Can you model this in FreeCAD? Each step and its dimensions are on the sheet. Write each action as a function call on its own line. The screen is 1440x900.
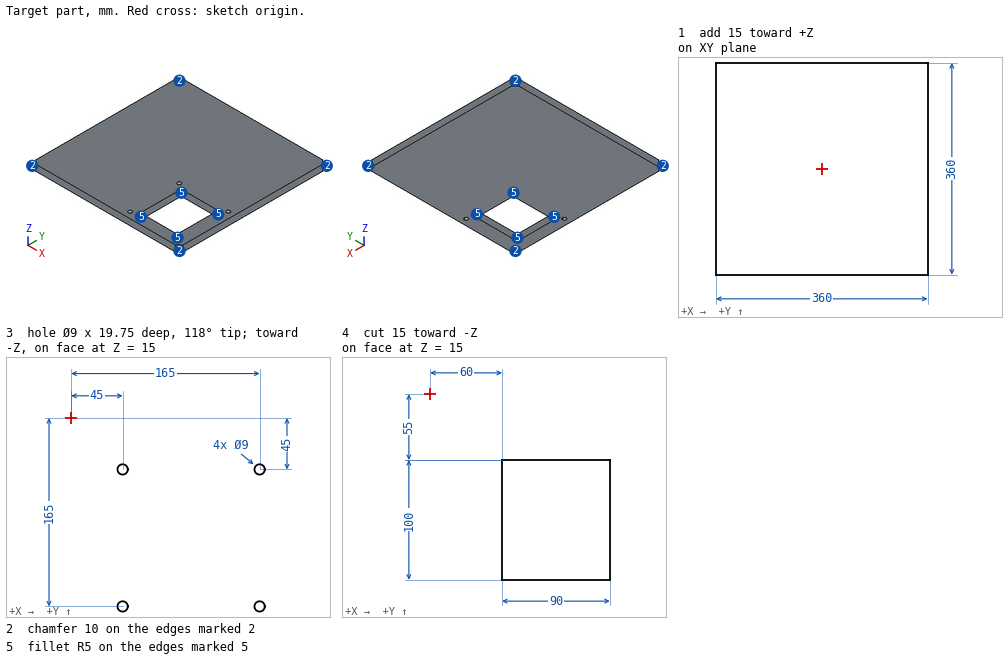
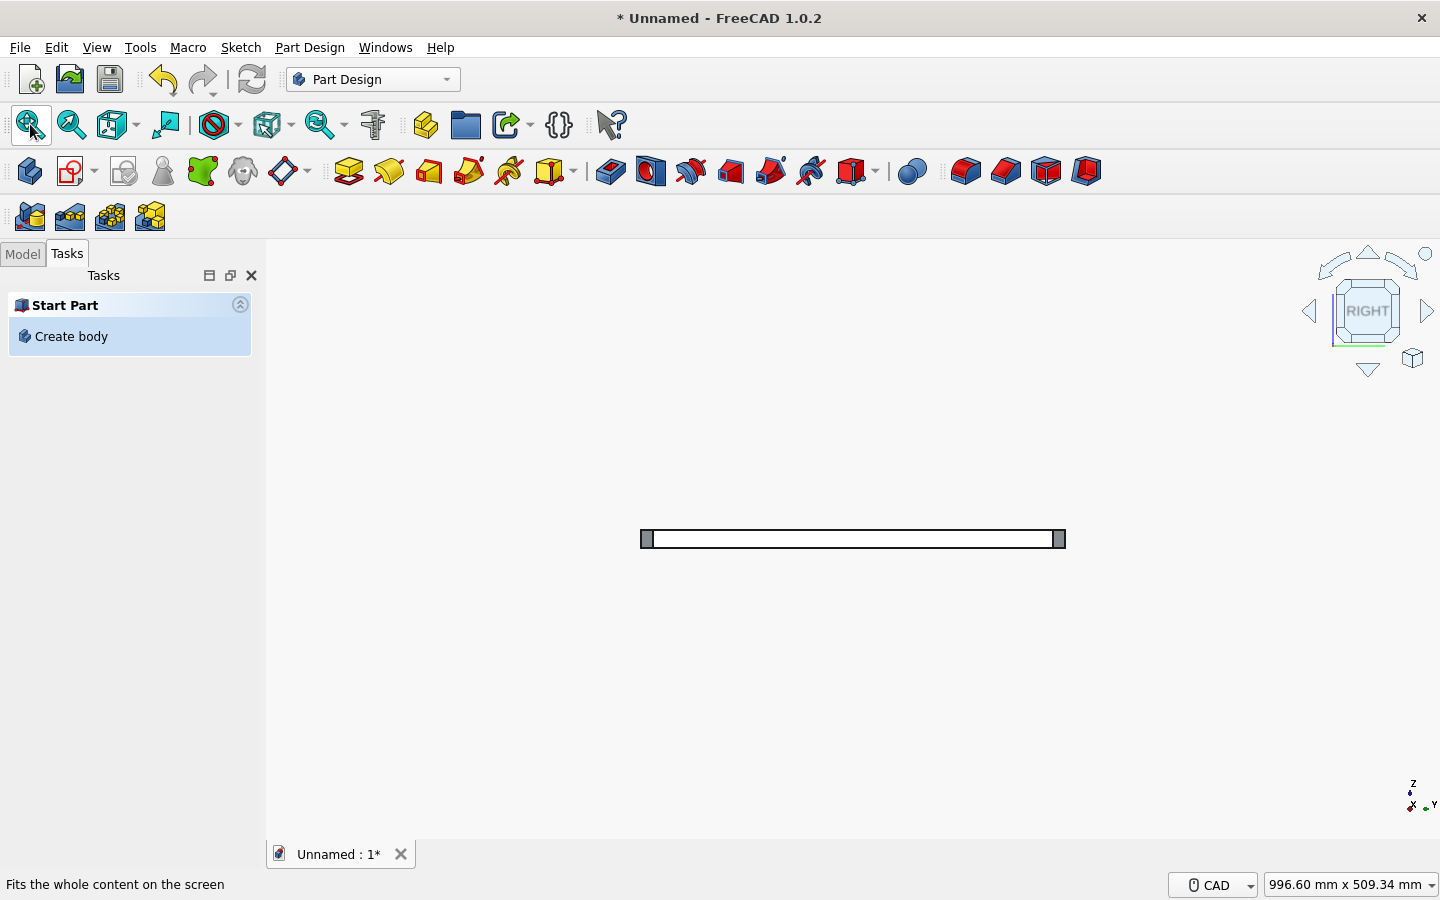
scroll(788, 538, up, 5)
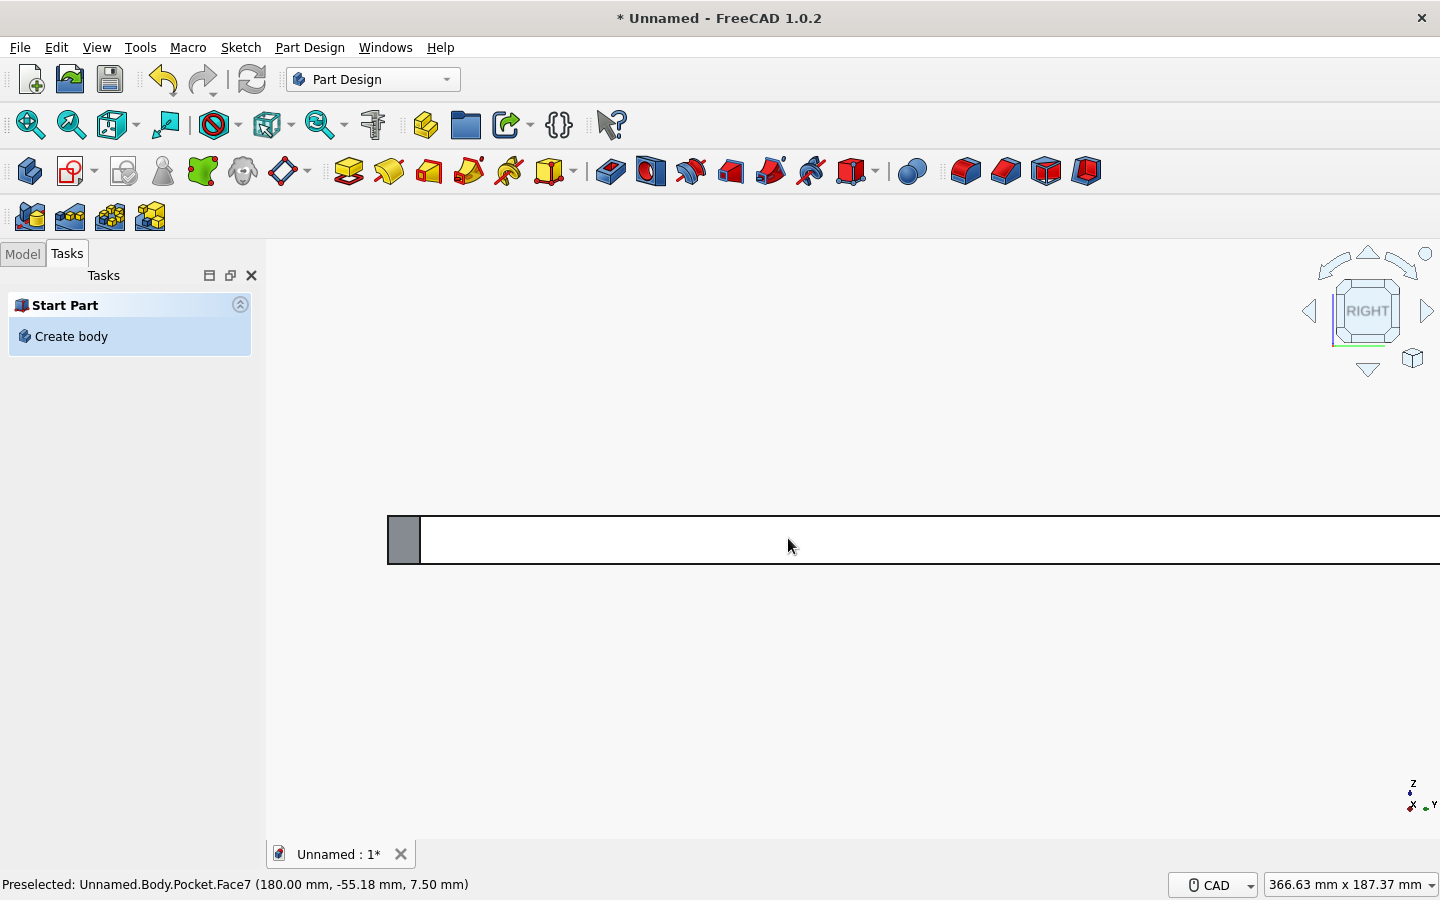
key(v)
key(f)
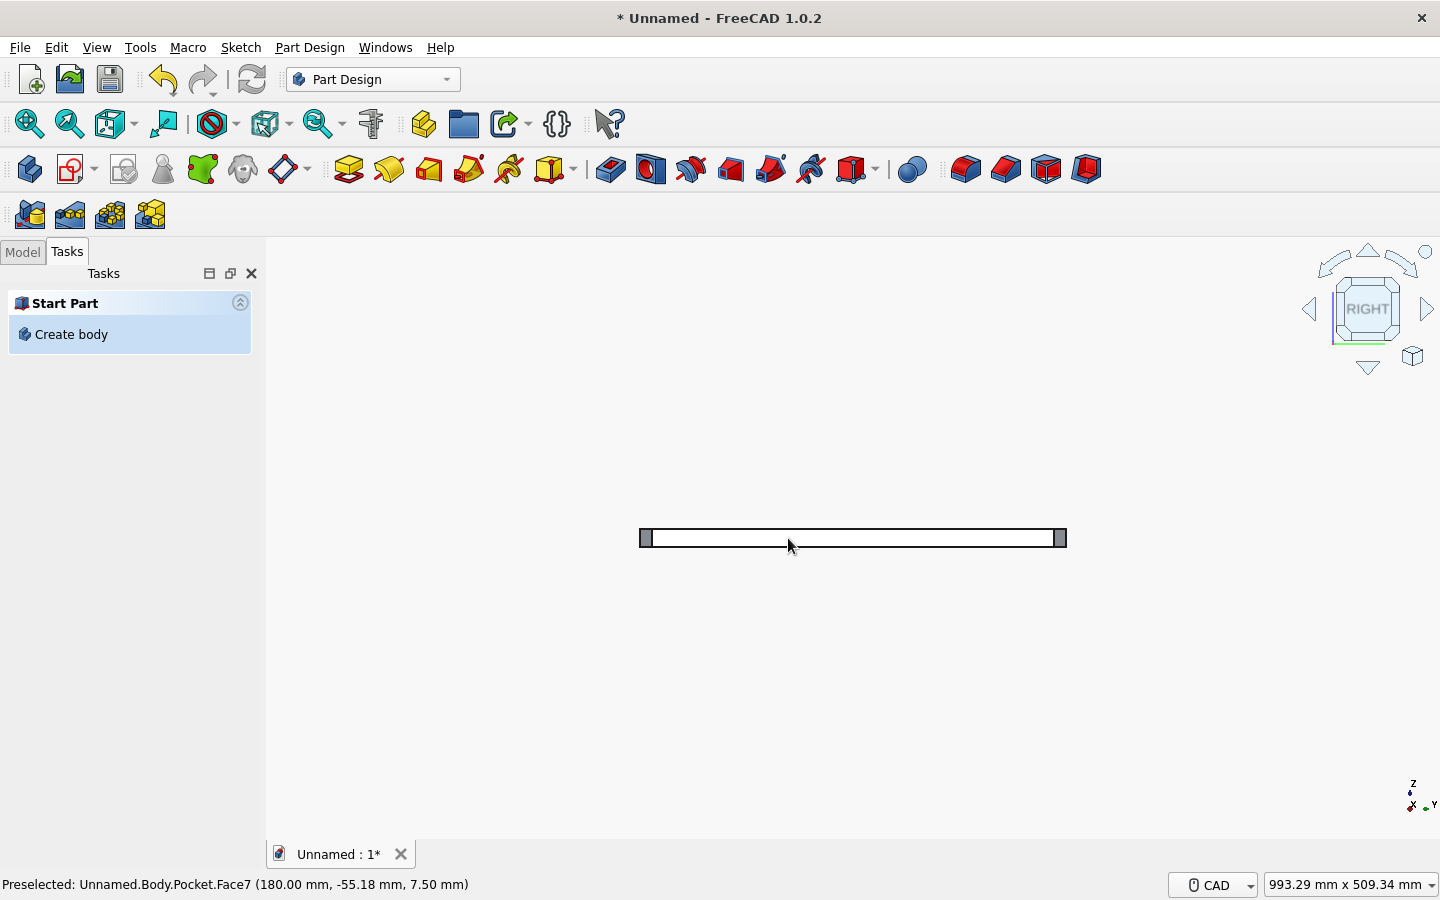
key(5)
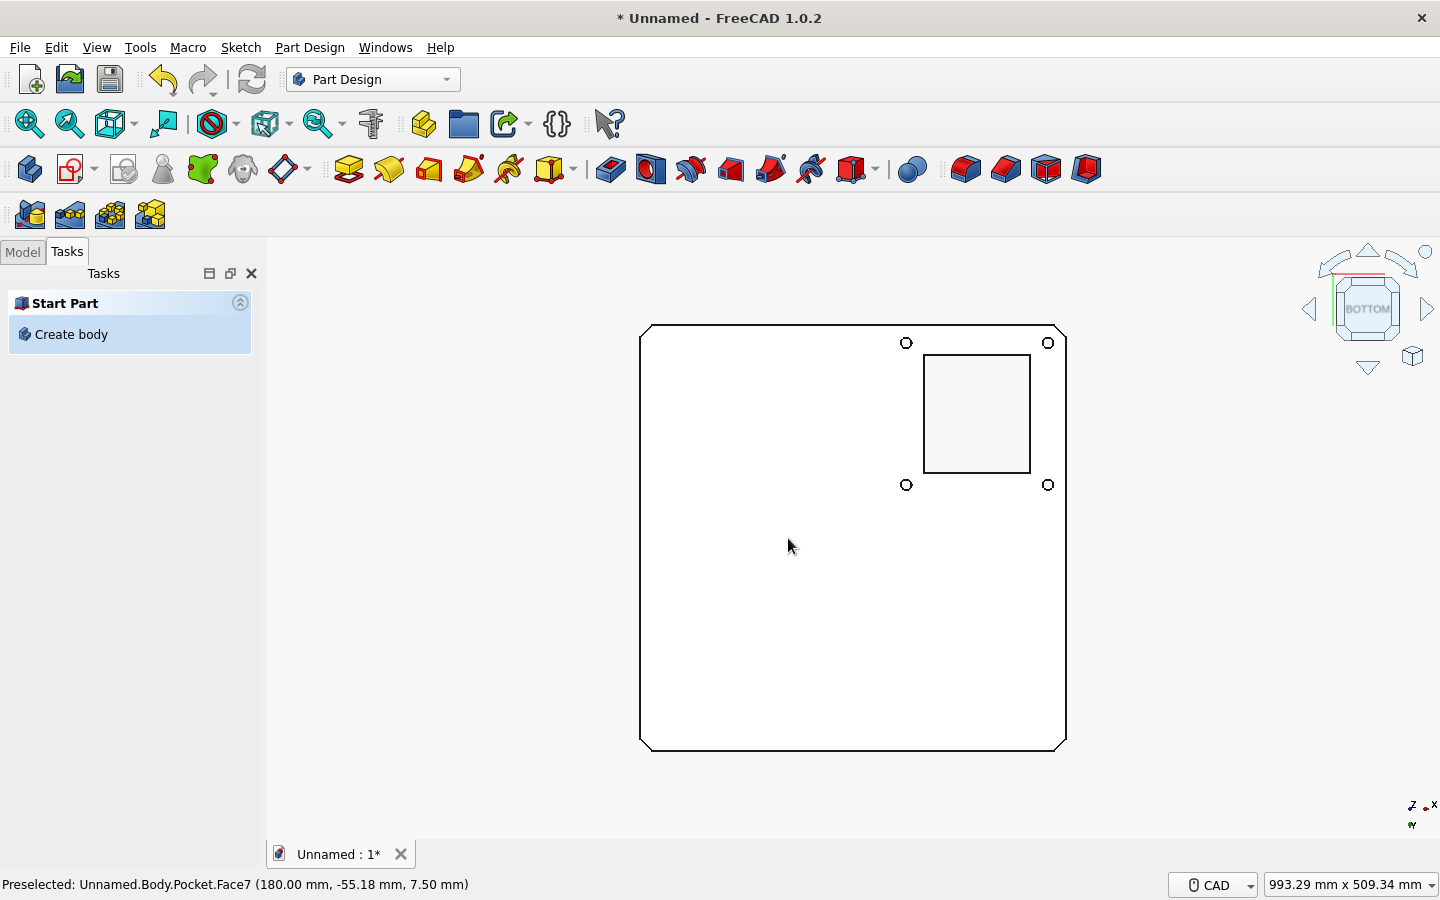
scroll(1030, 472, up, 5)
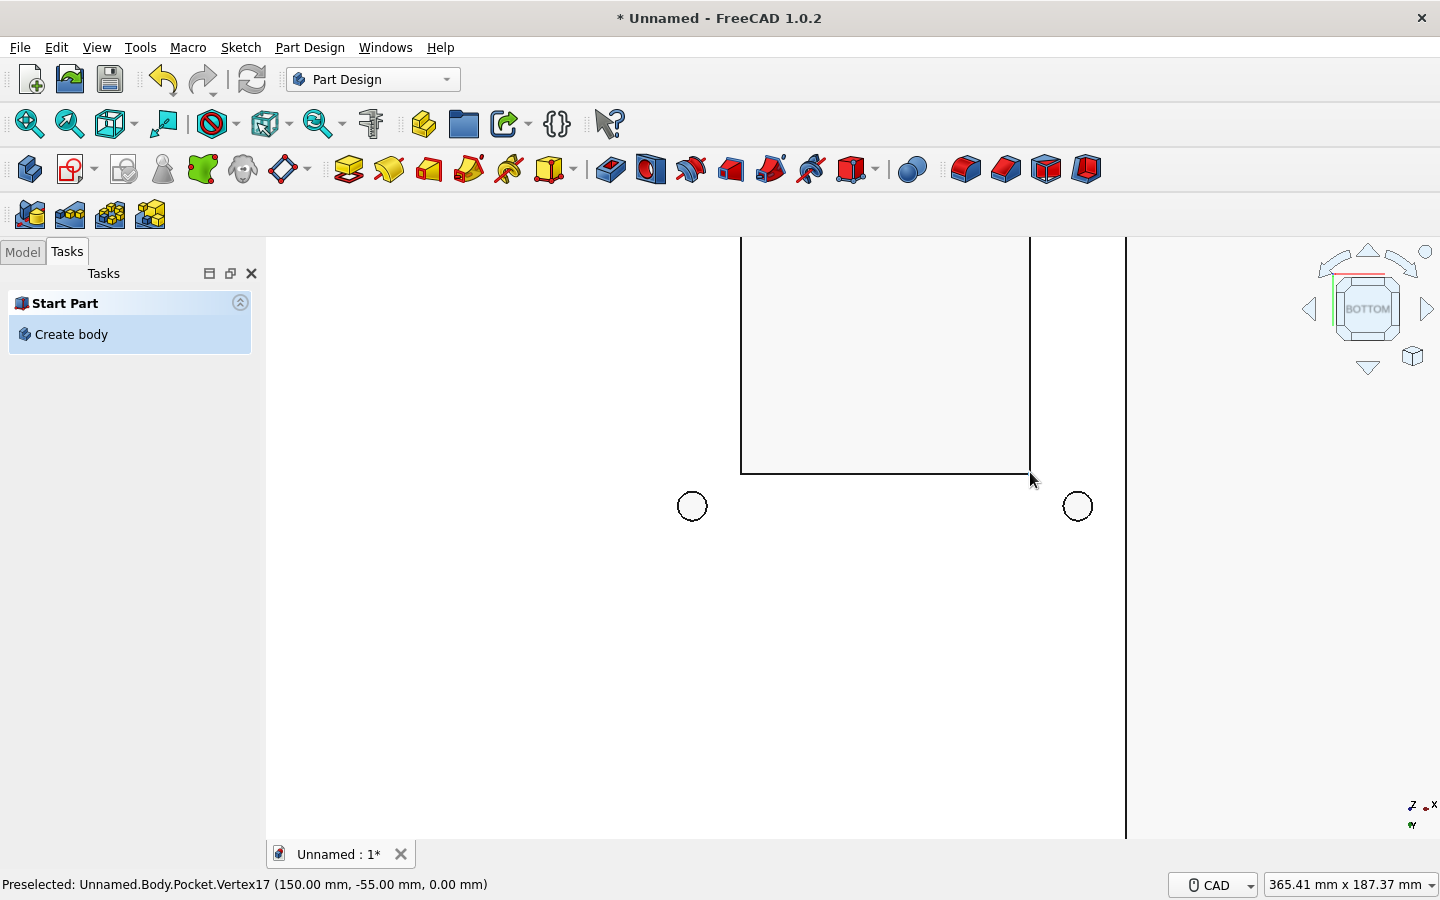
key(v)
key(f)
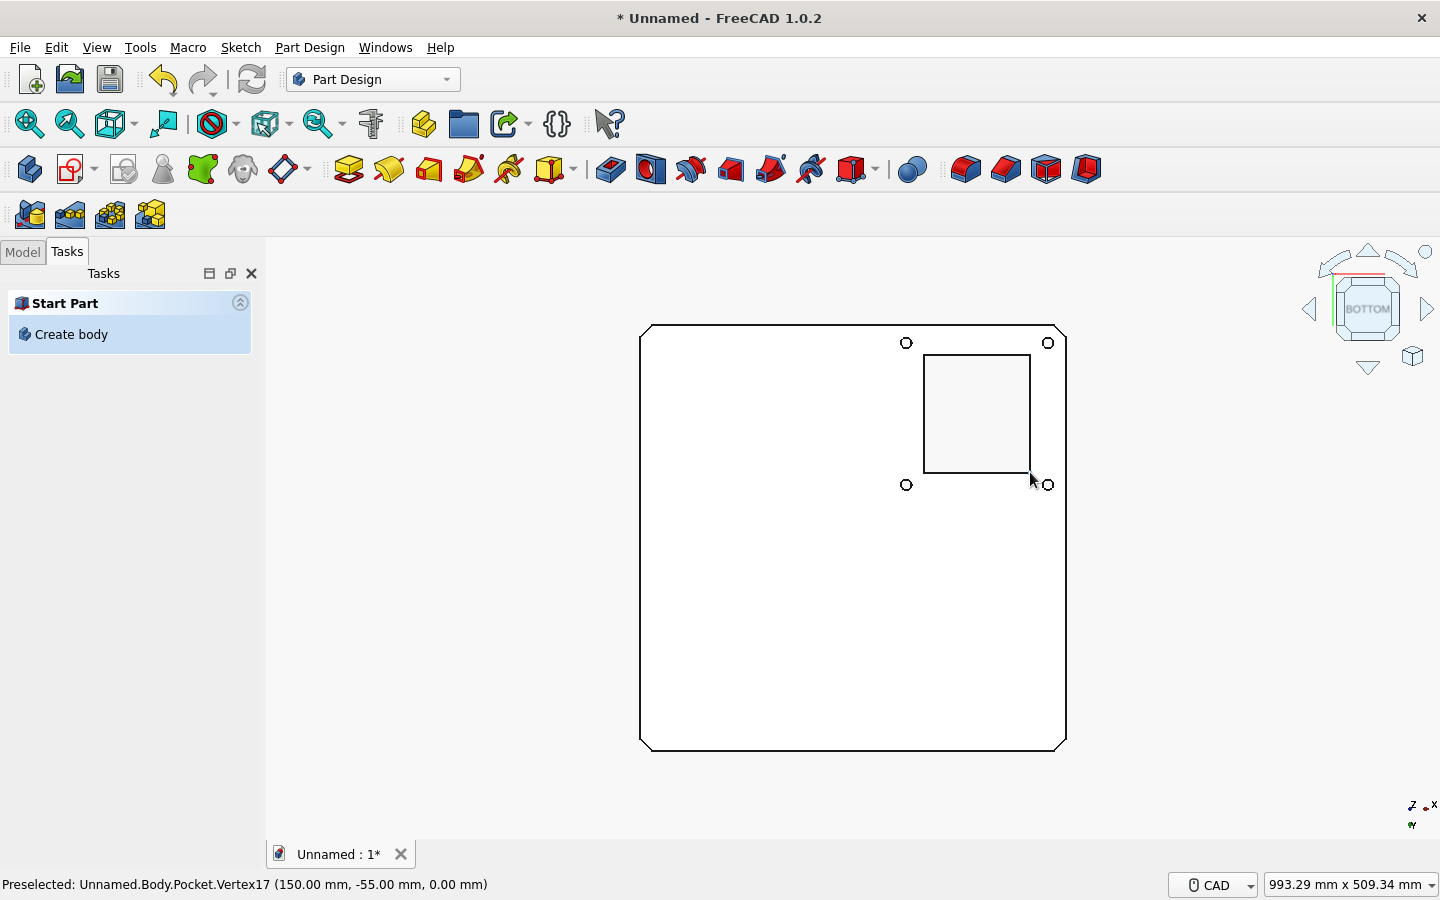
key(4)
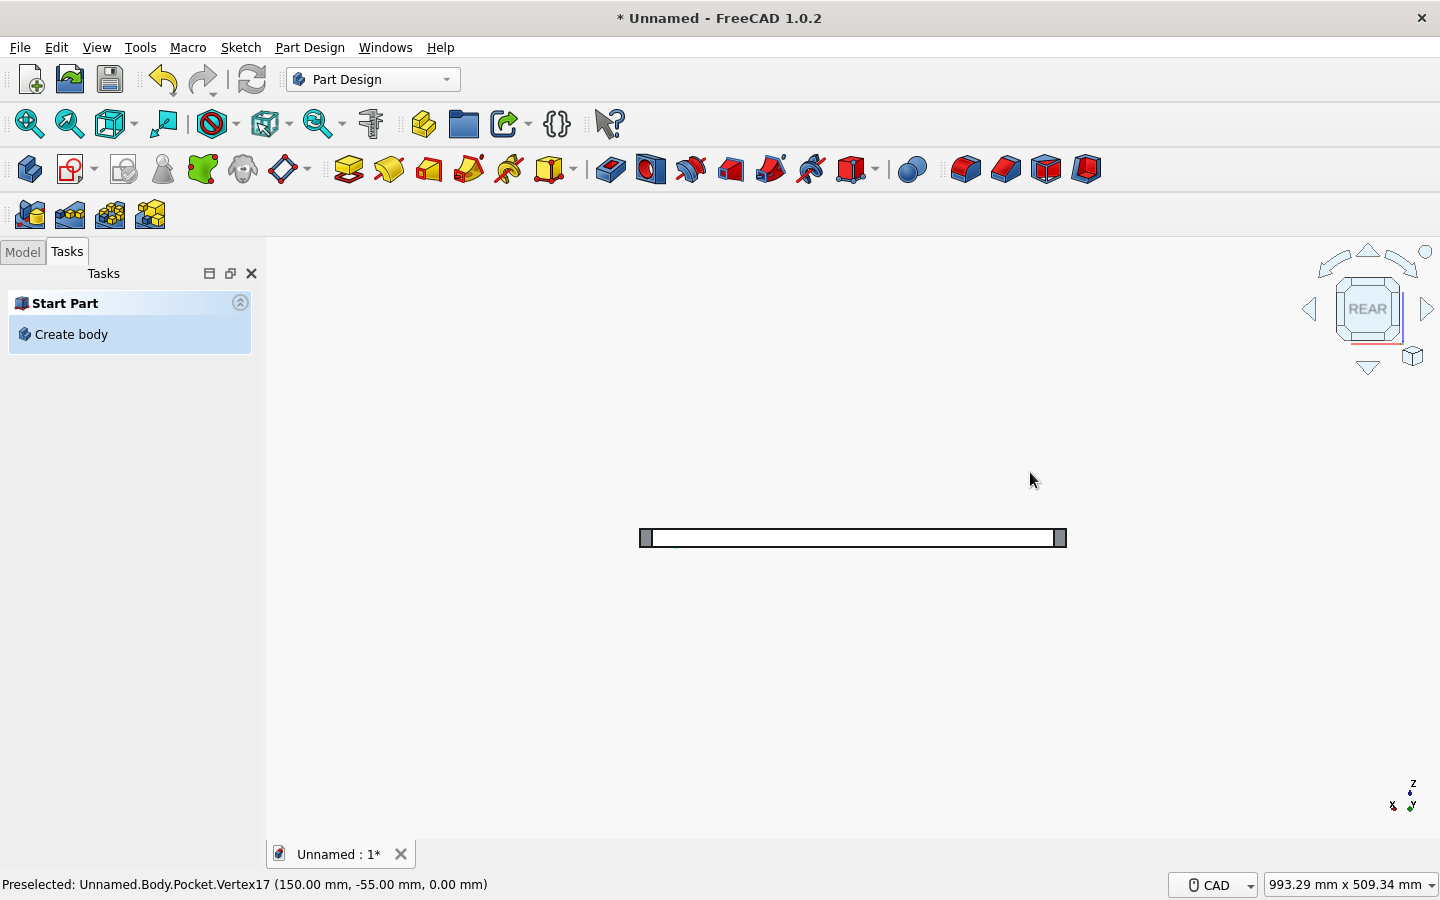
key(v)
key(f)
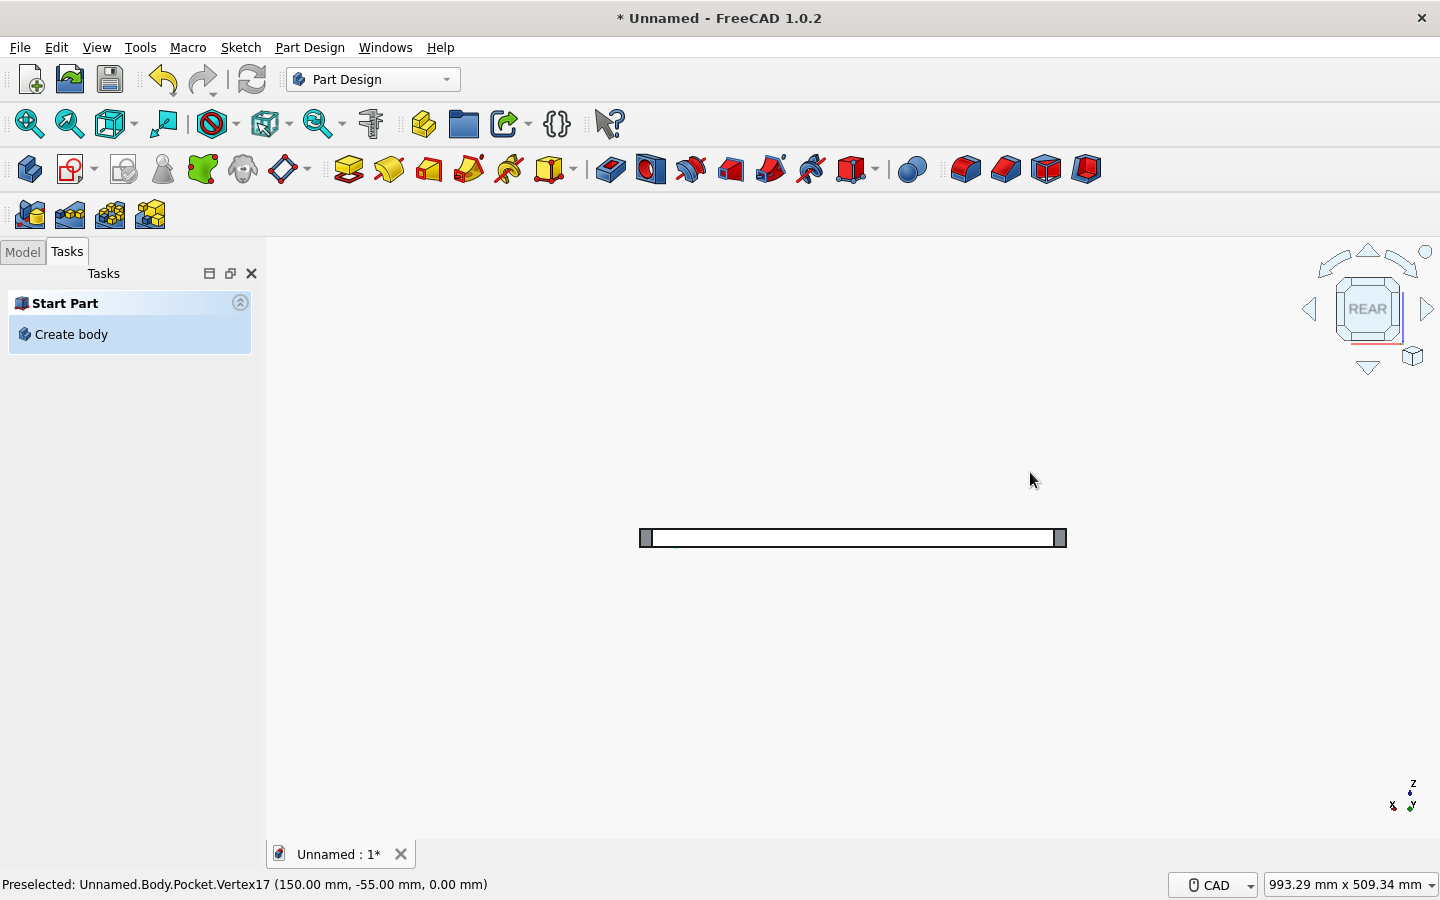
scroll(676, 537, up, 5)